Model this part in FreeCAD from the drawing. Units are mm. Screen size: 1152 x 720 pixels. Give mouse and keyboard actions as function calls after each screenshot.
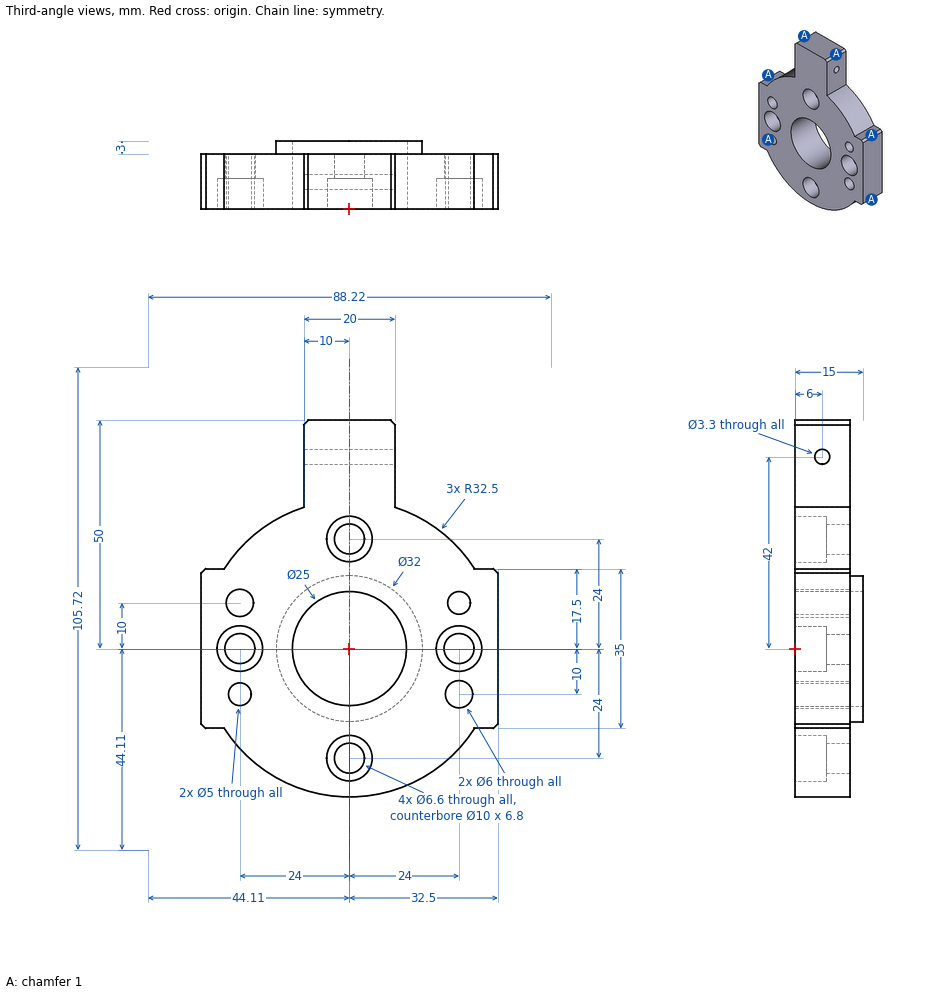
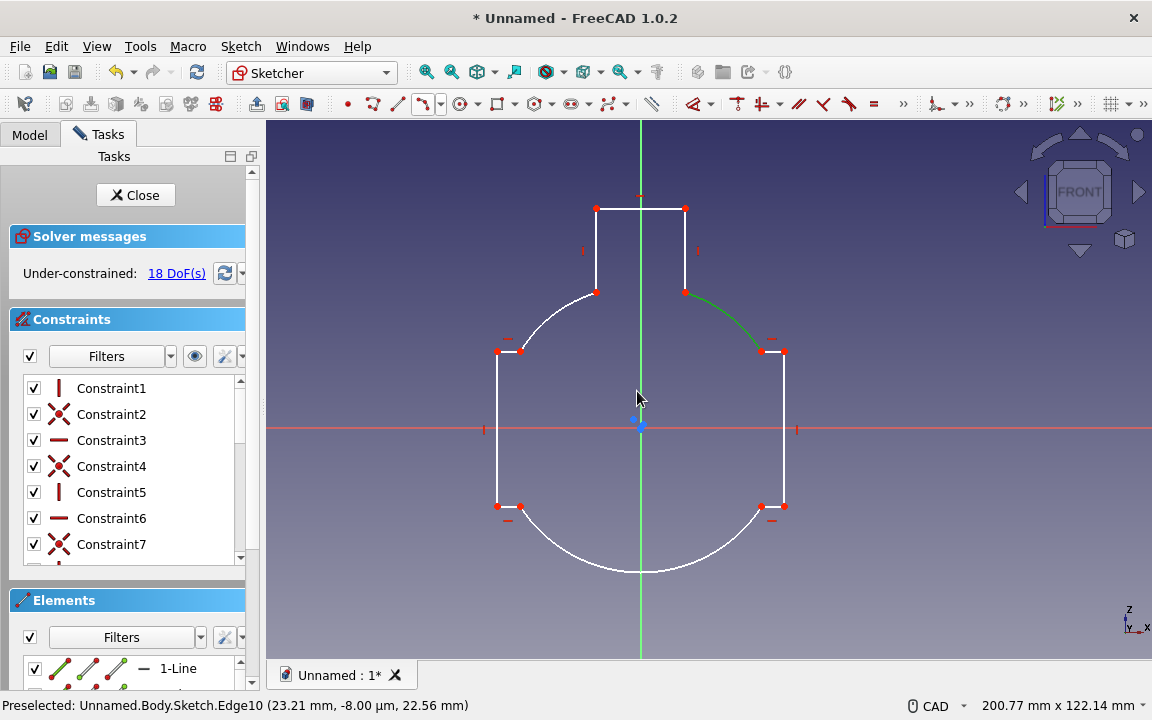
click(585, 561)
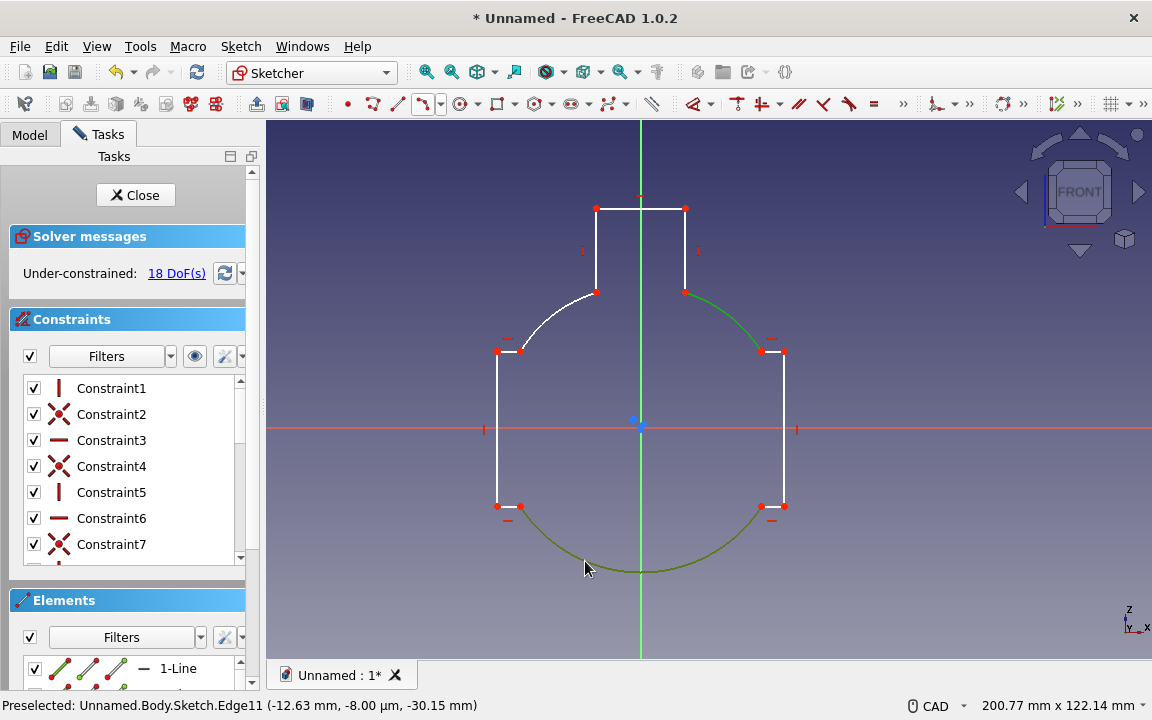
click(737, 104)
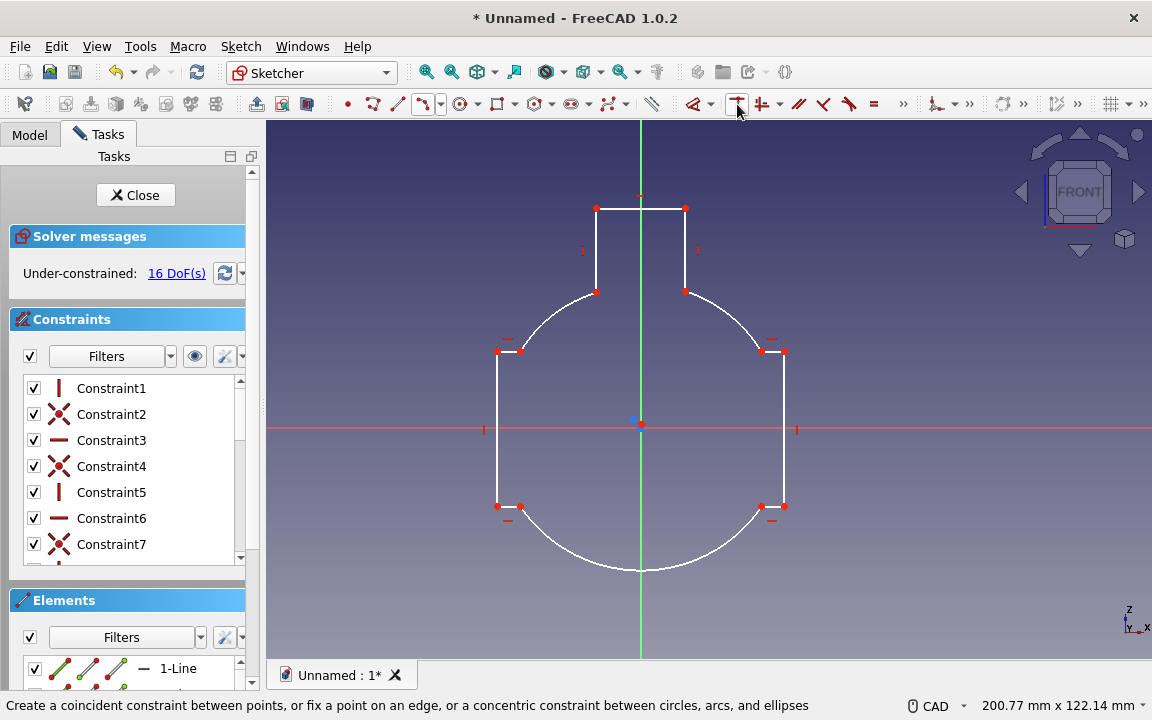
click(743, 328)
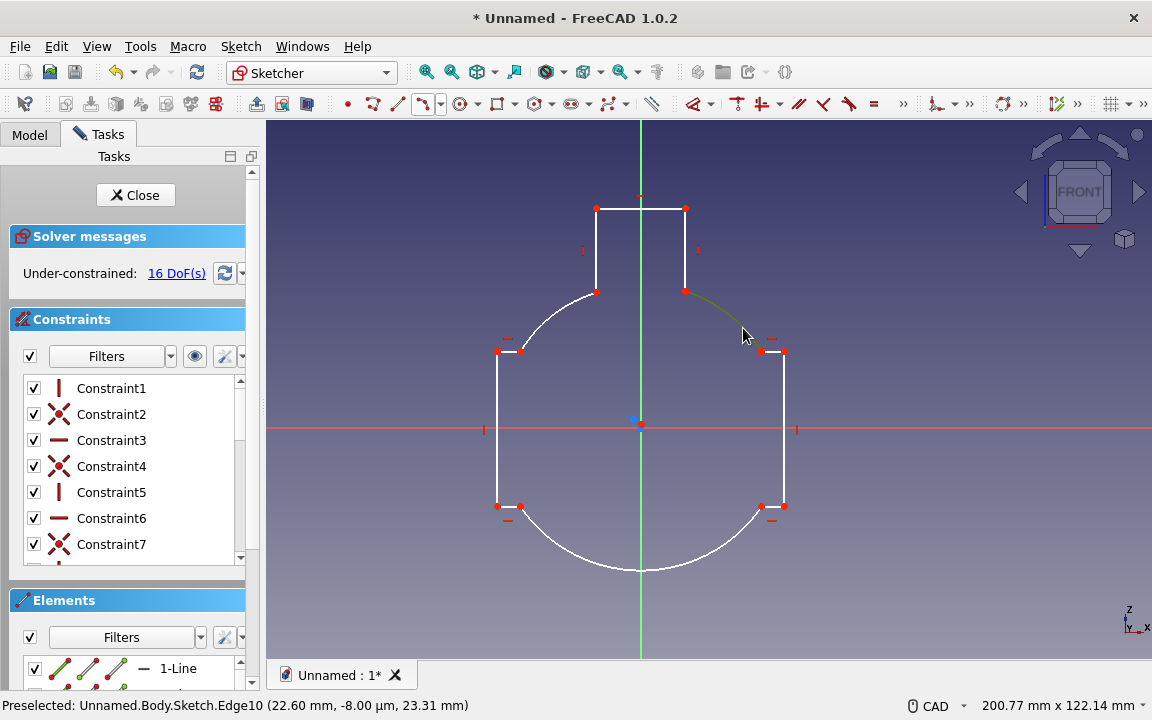
click(569, 304)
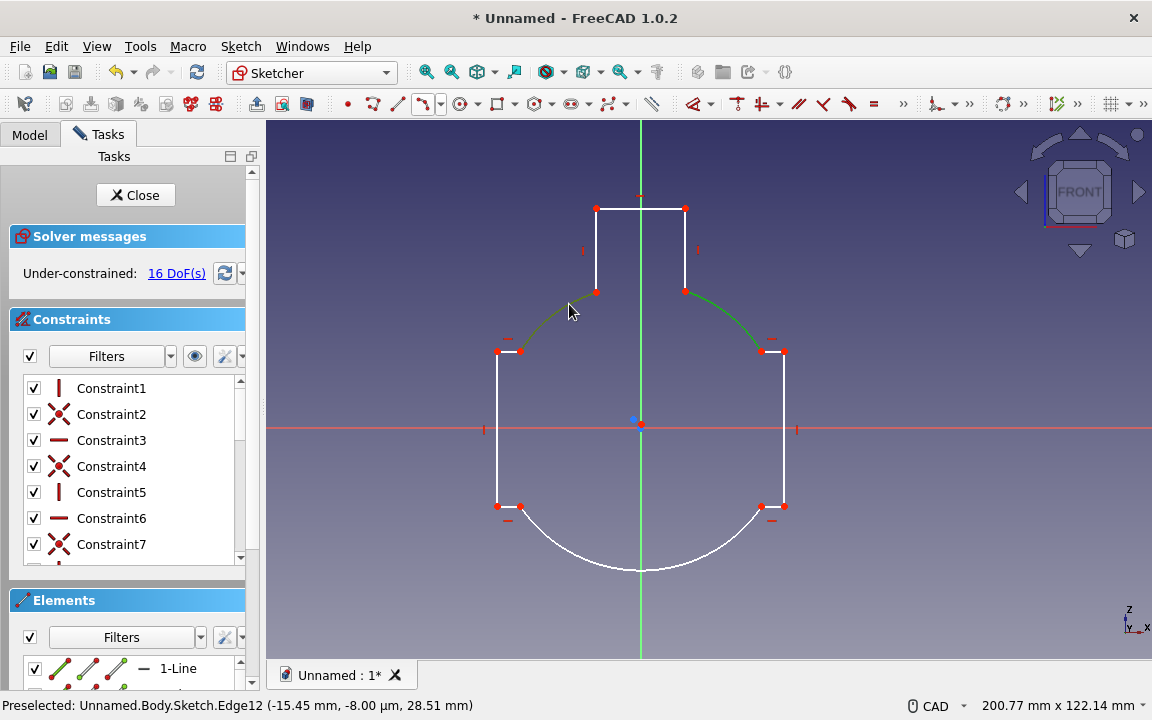
click(737, 104)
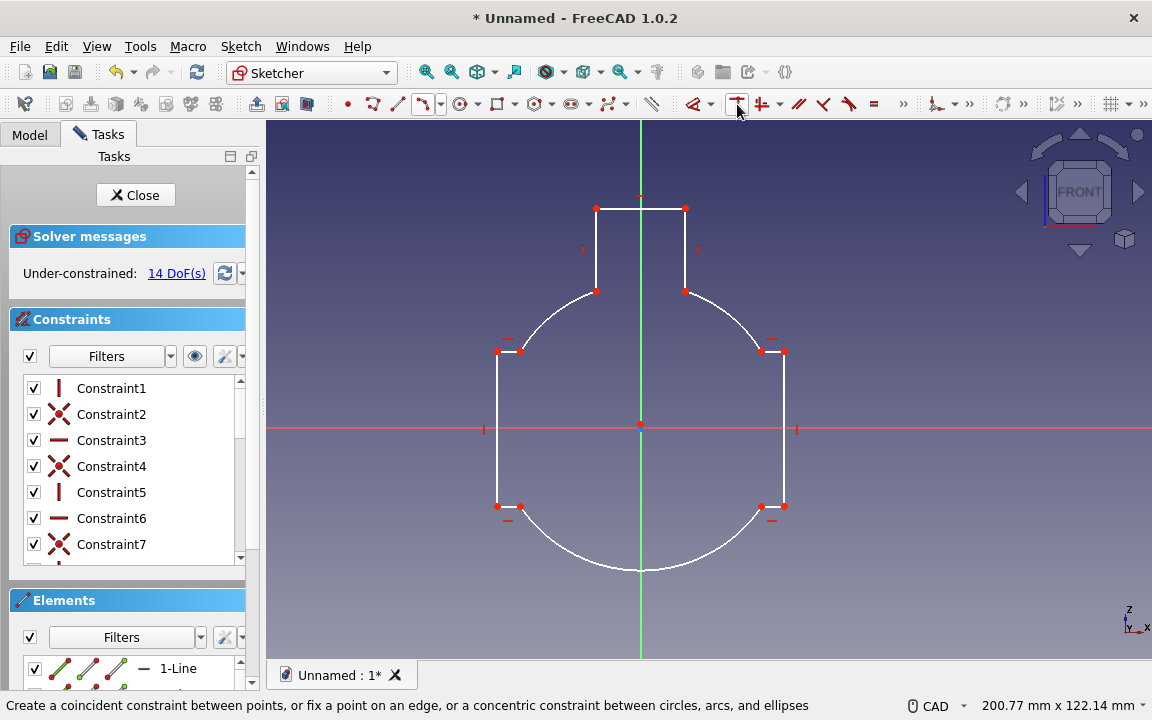
drag(631, 415, 651, 438)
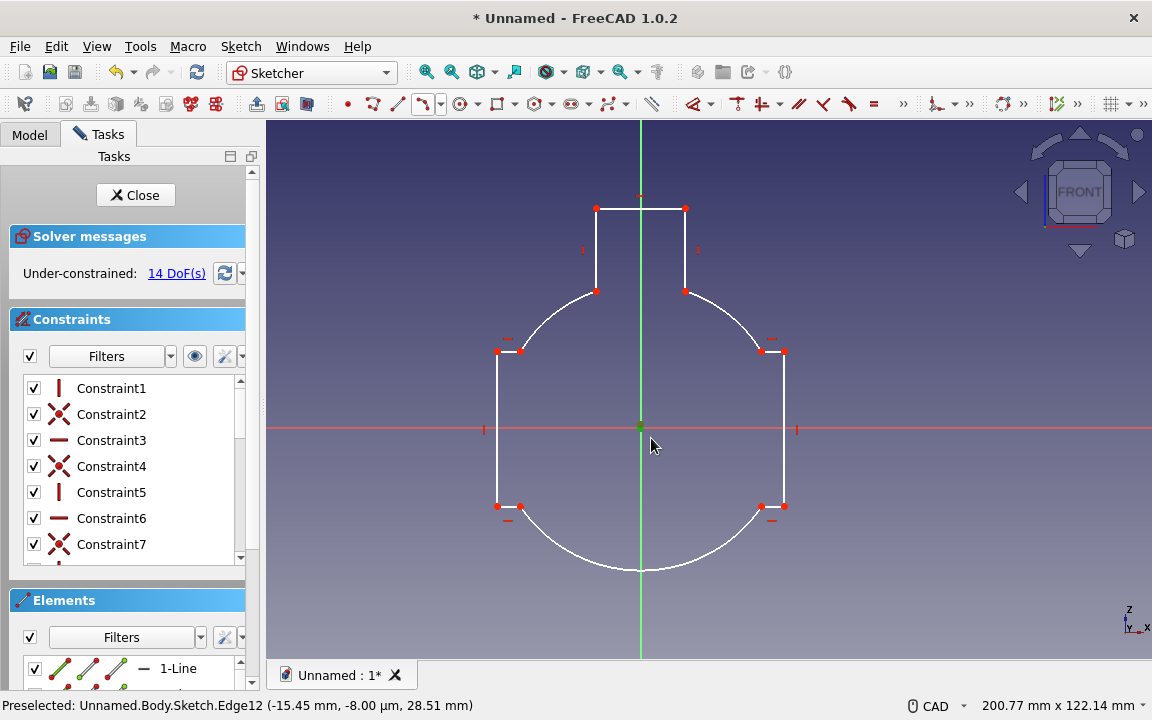
click(737, 104)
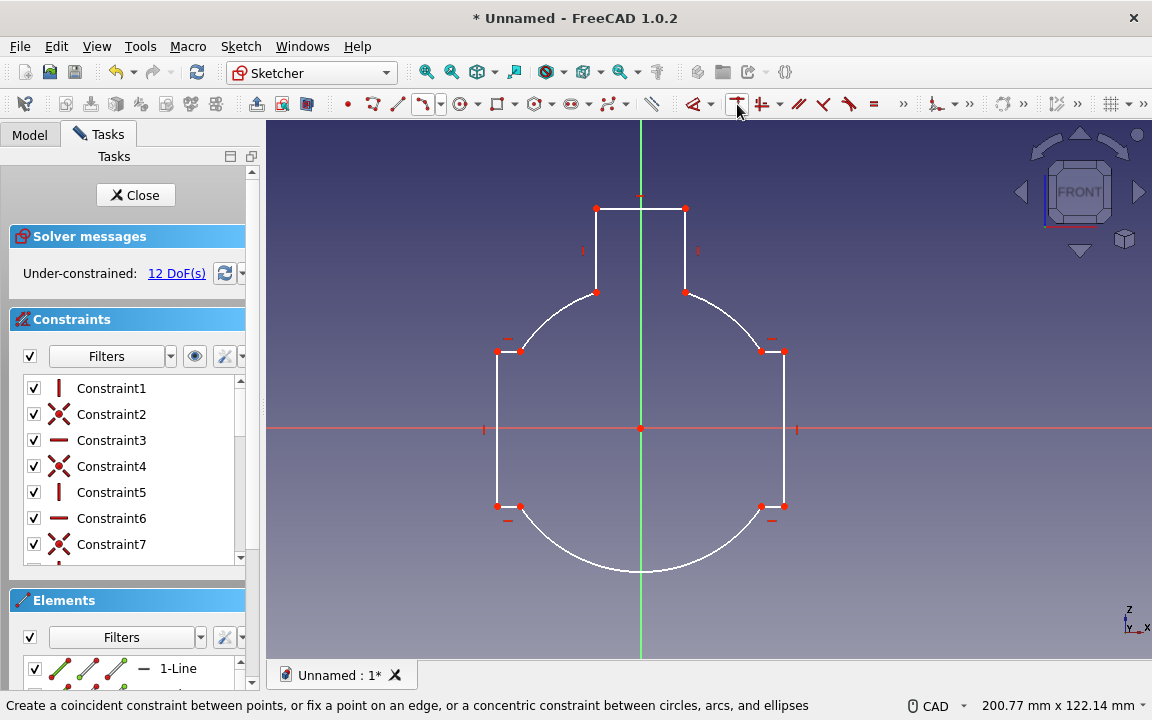
click(743, 329)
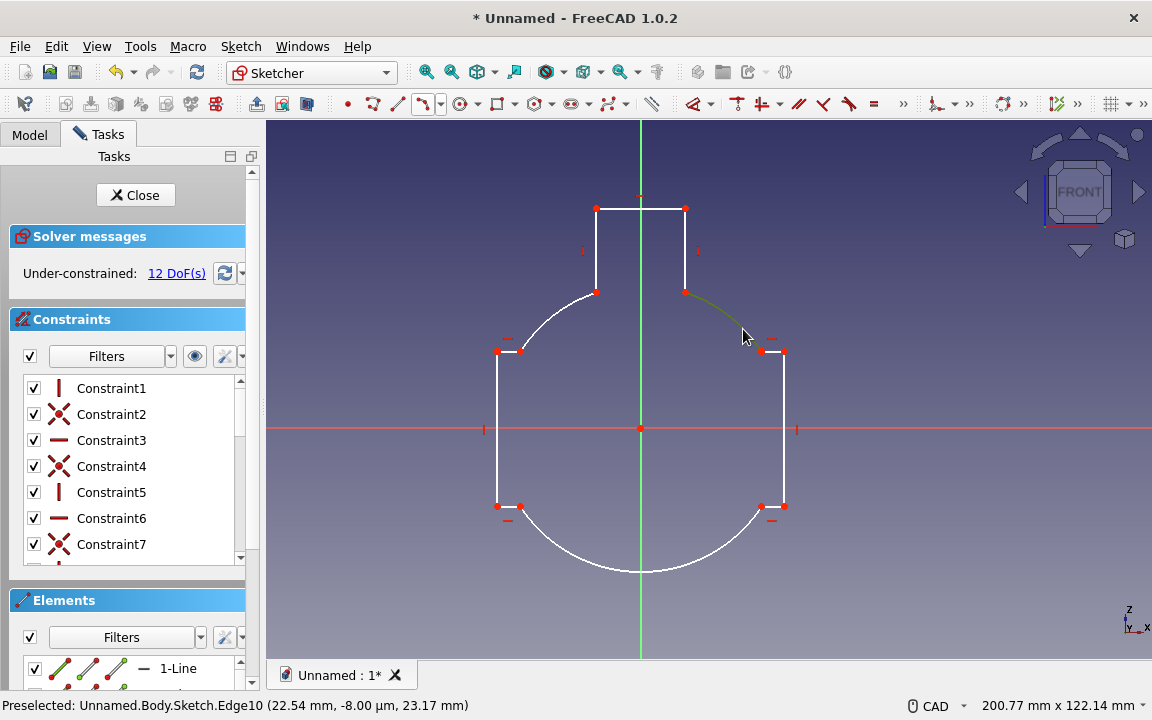
click(585, 561)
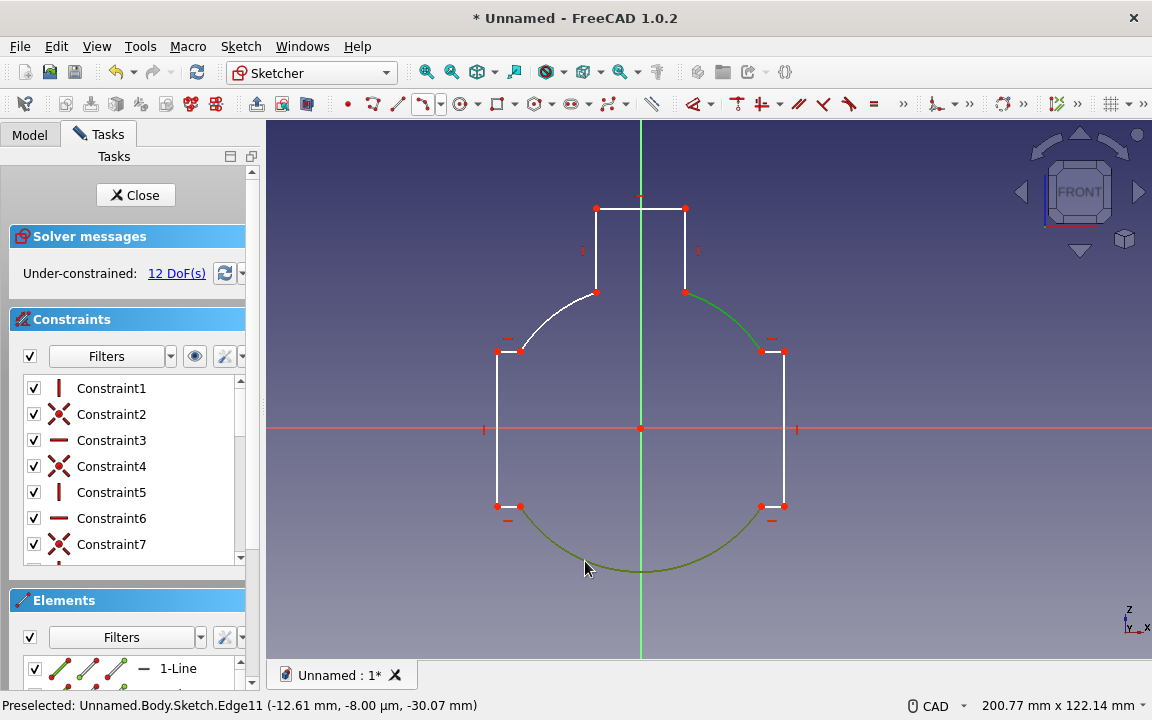
click(570, 305)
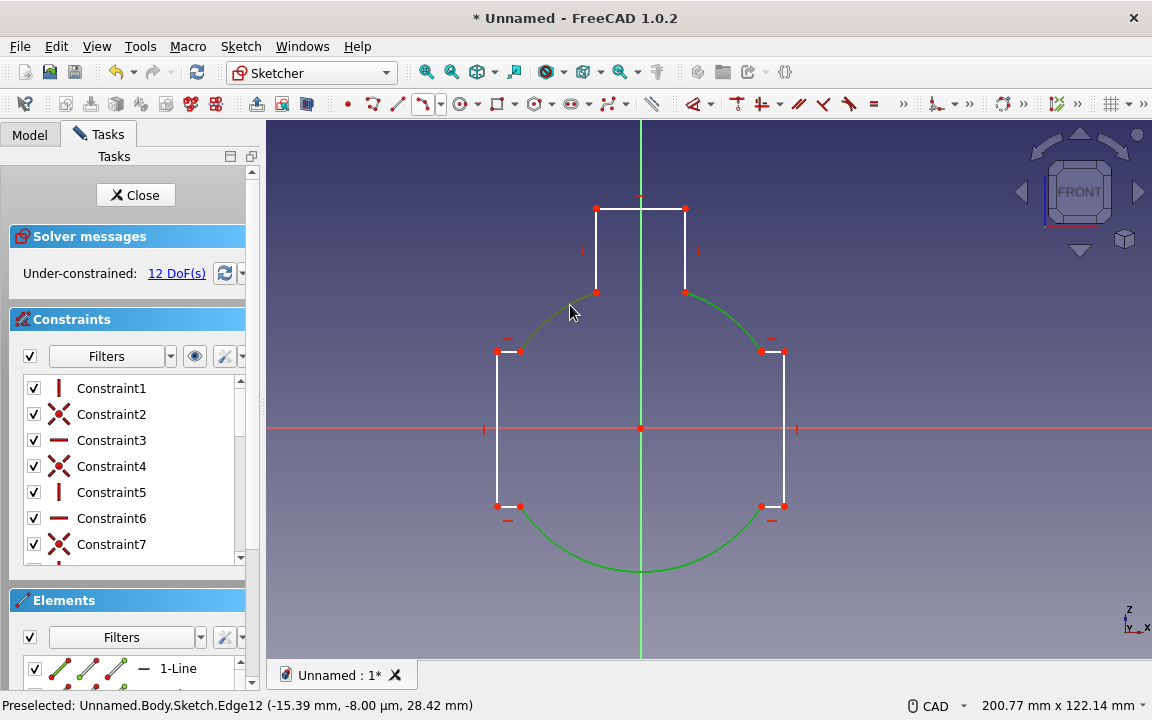
click(874, 104)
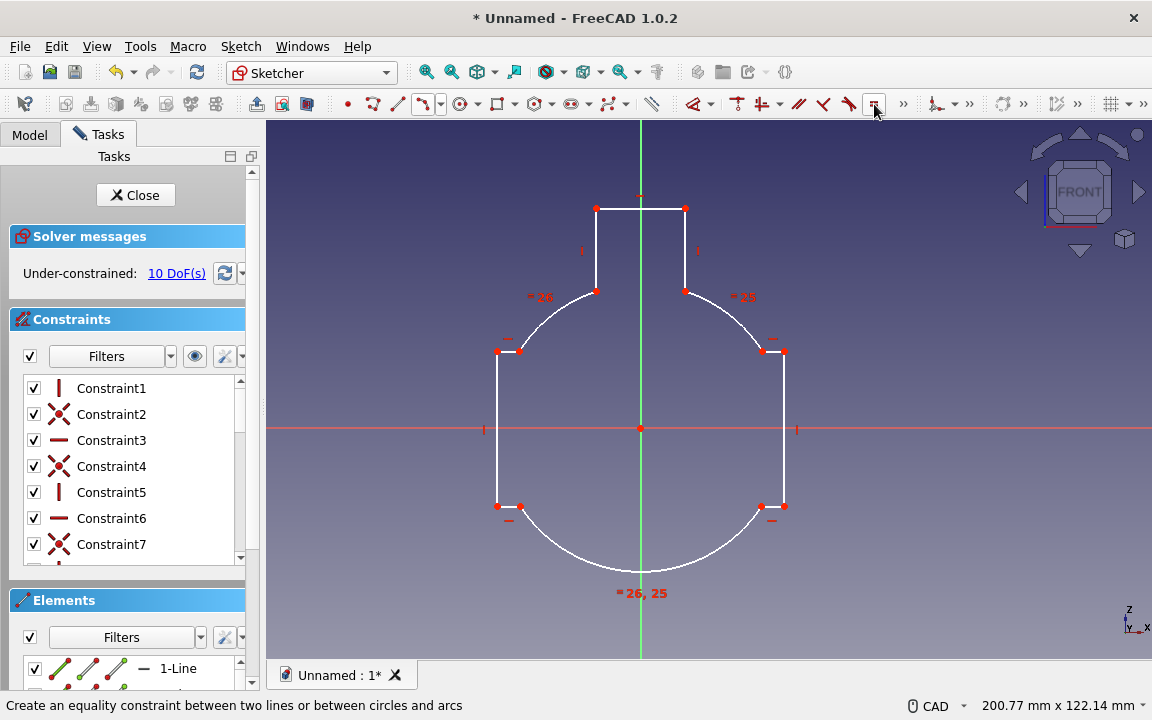
click(784, 507)